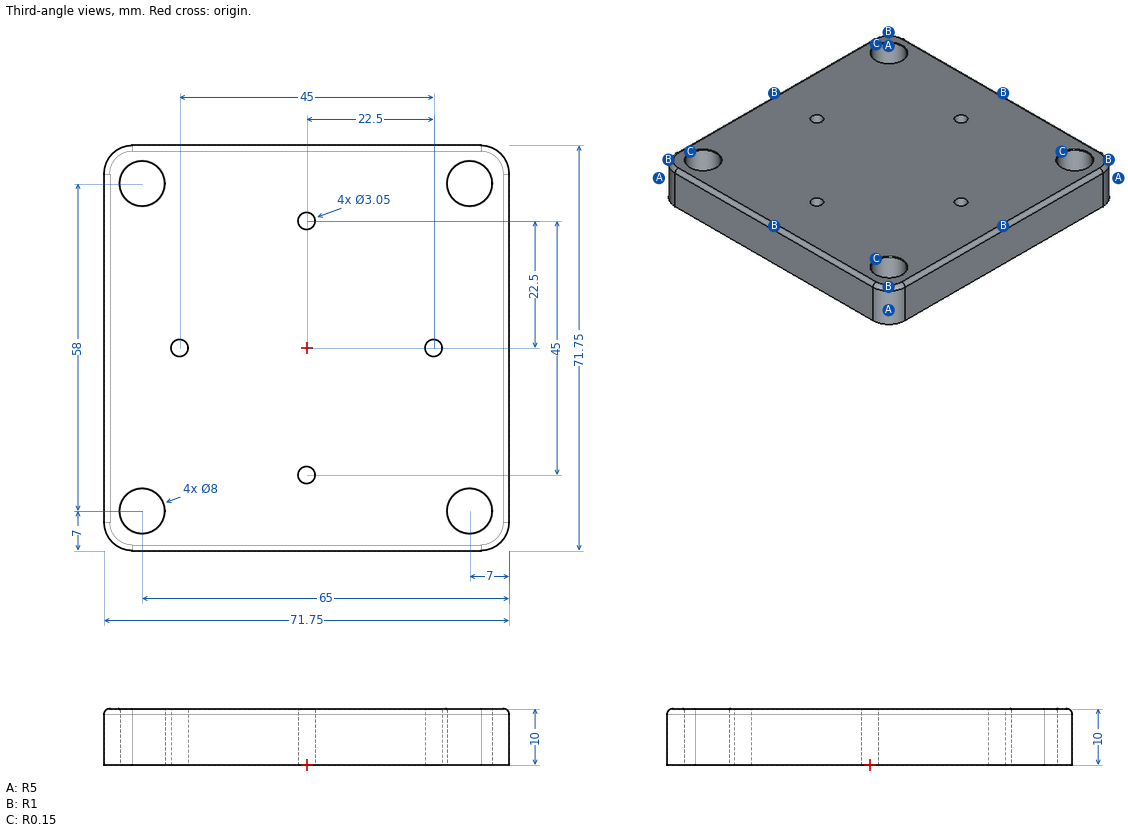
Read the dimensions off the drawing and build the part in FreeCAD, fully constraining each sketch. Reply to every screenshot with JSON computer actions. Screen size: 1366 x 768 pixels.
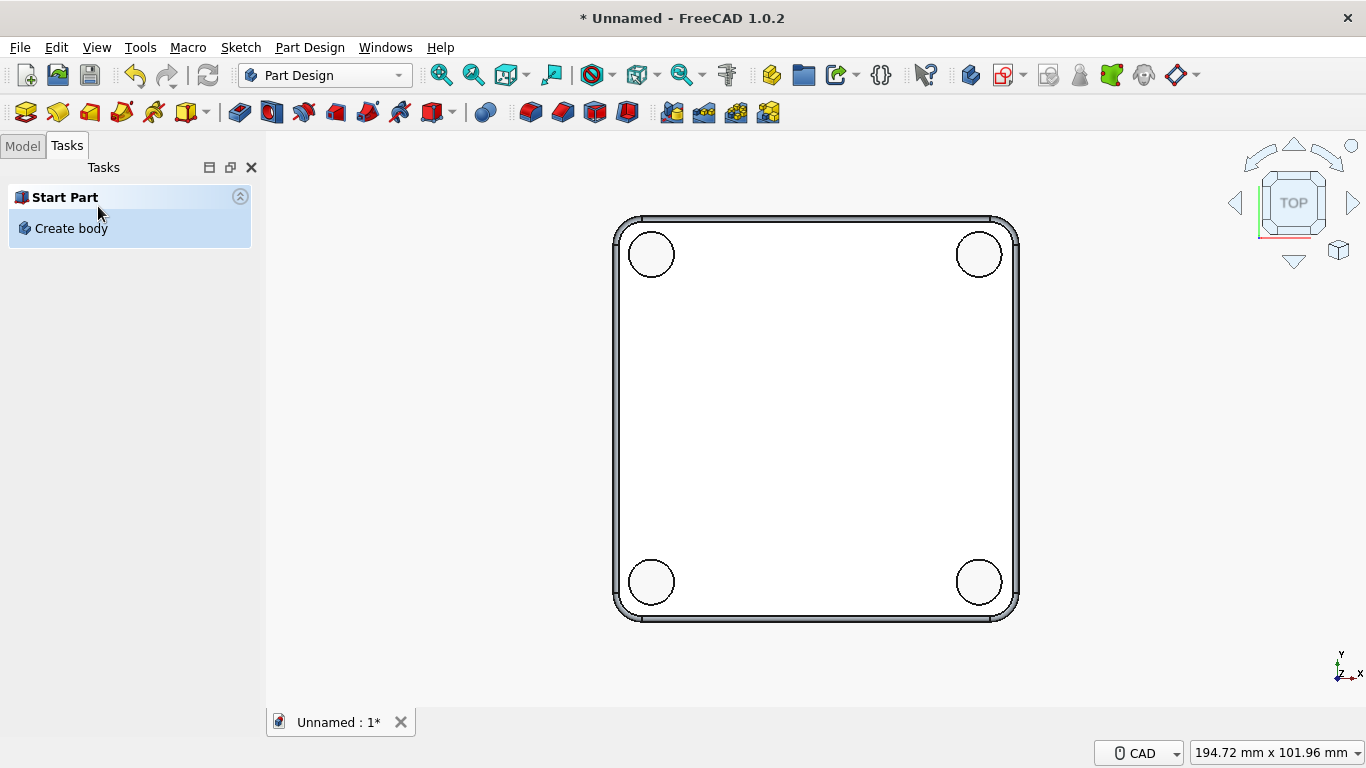
{"action": "left_click", "coordinate": [629, 253]}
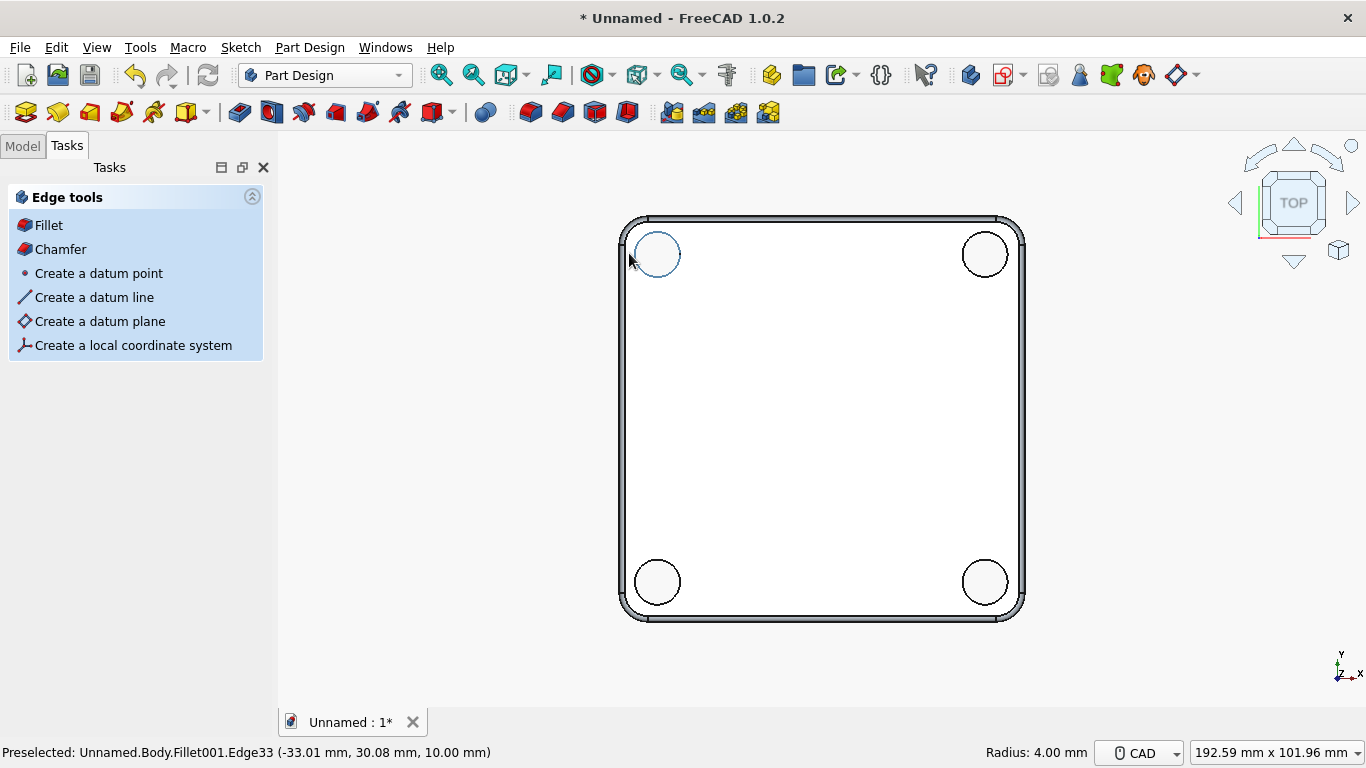
{"action": "left_click", "coordinate": [963, 253], "text": "ctrl"}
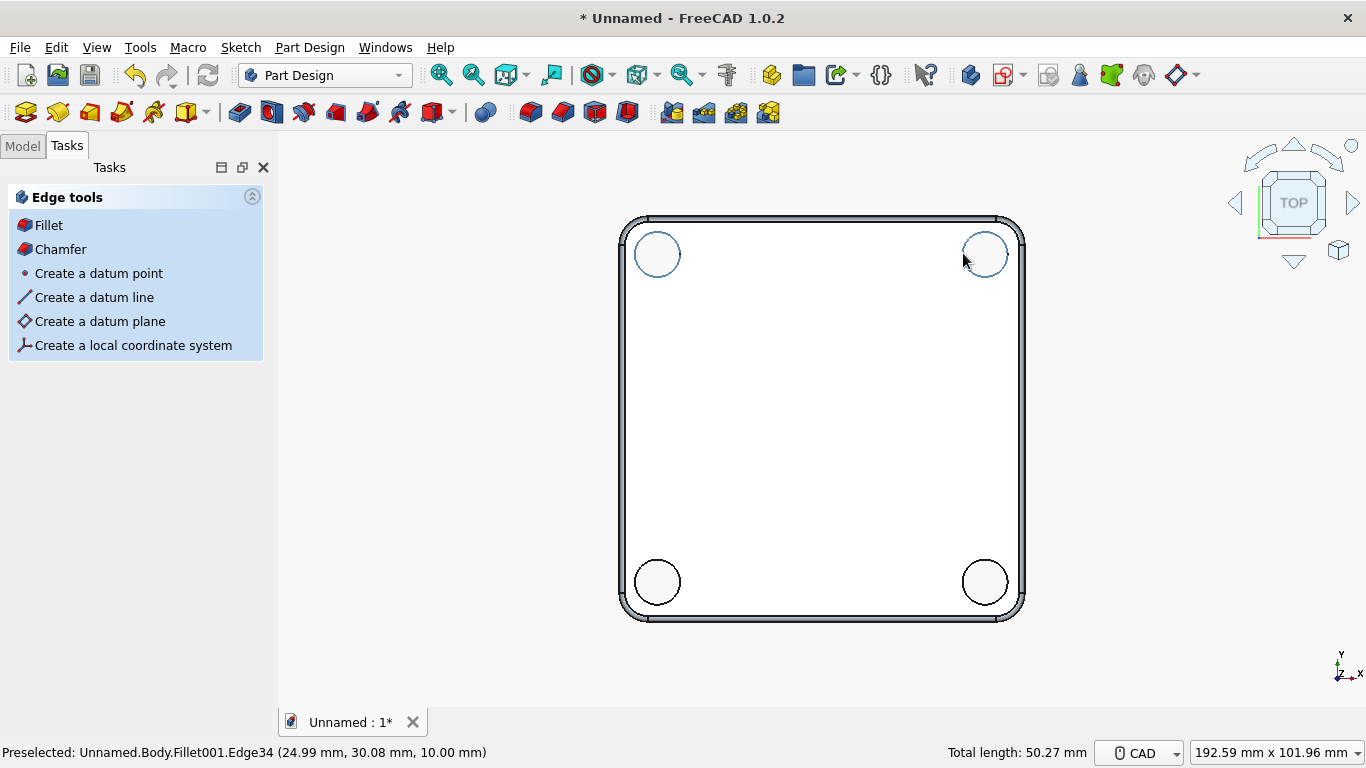
{"action": "left_click", "coordinate": [963, 581], "text": "ctrl"}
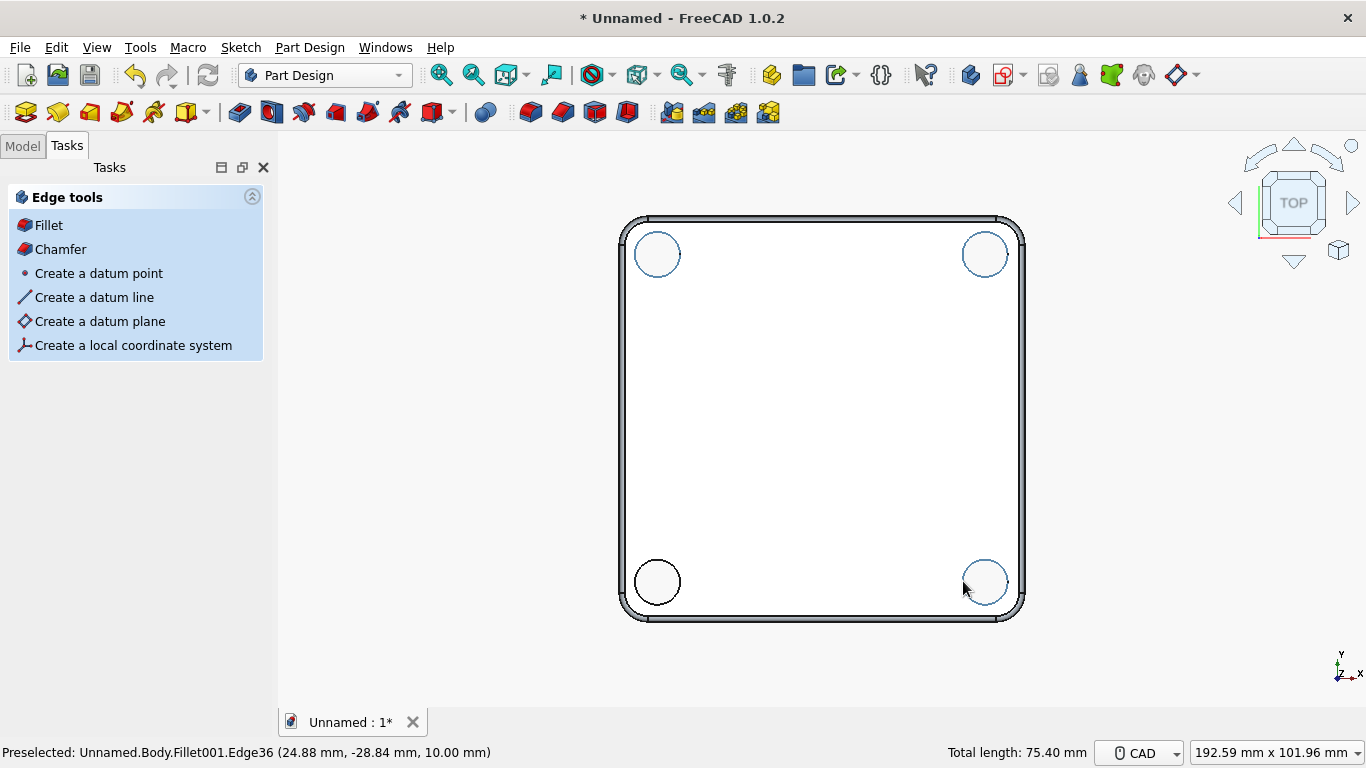
{"action": "left_click", "coordinate": [635, 581], "text": "ctrl"}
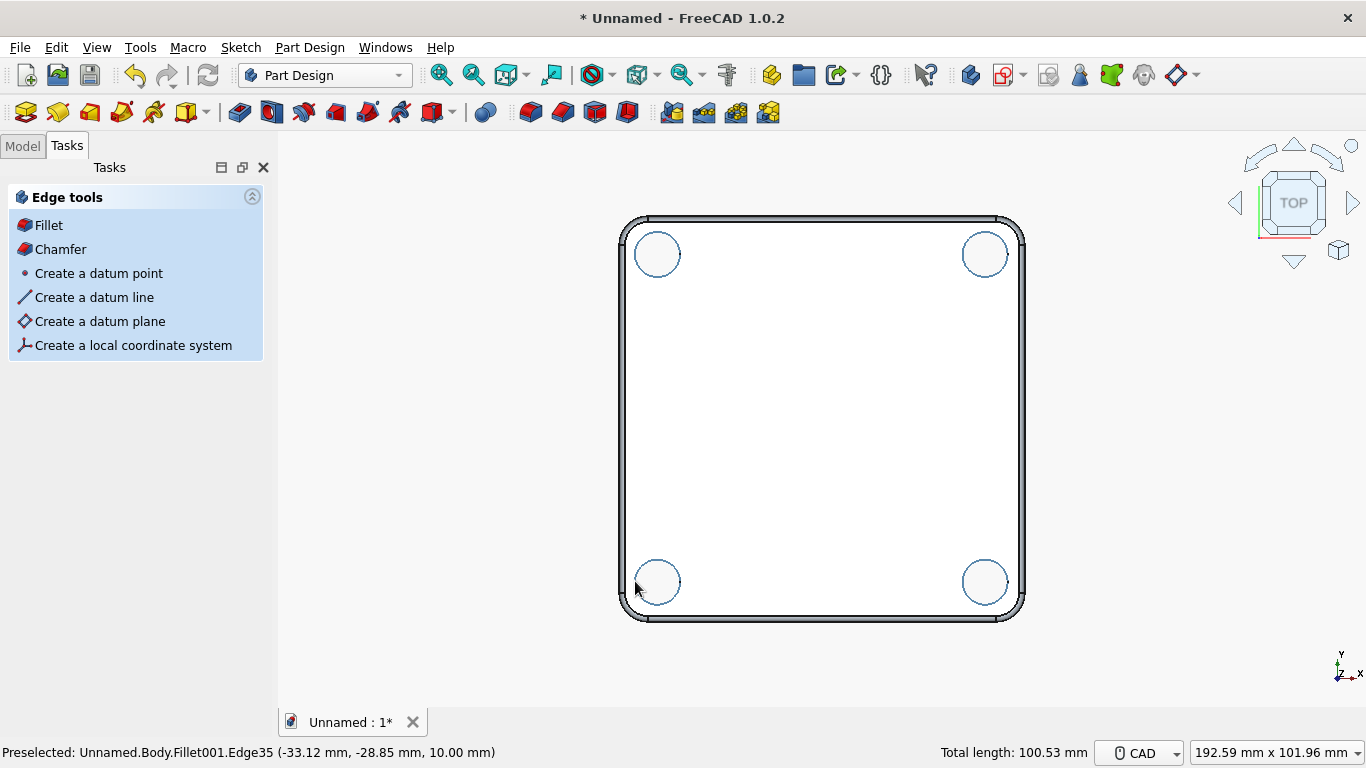
{"action": "left_click", "coordinate": [532, 112]}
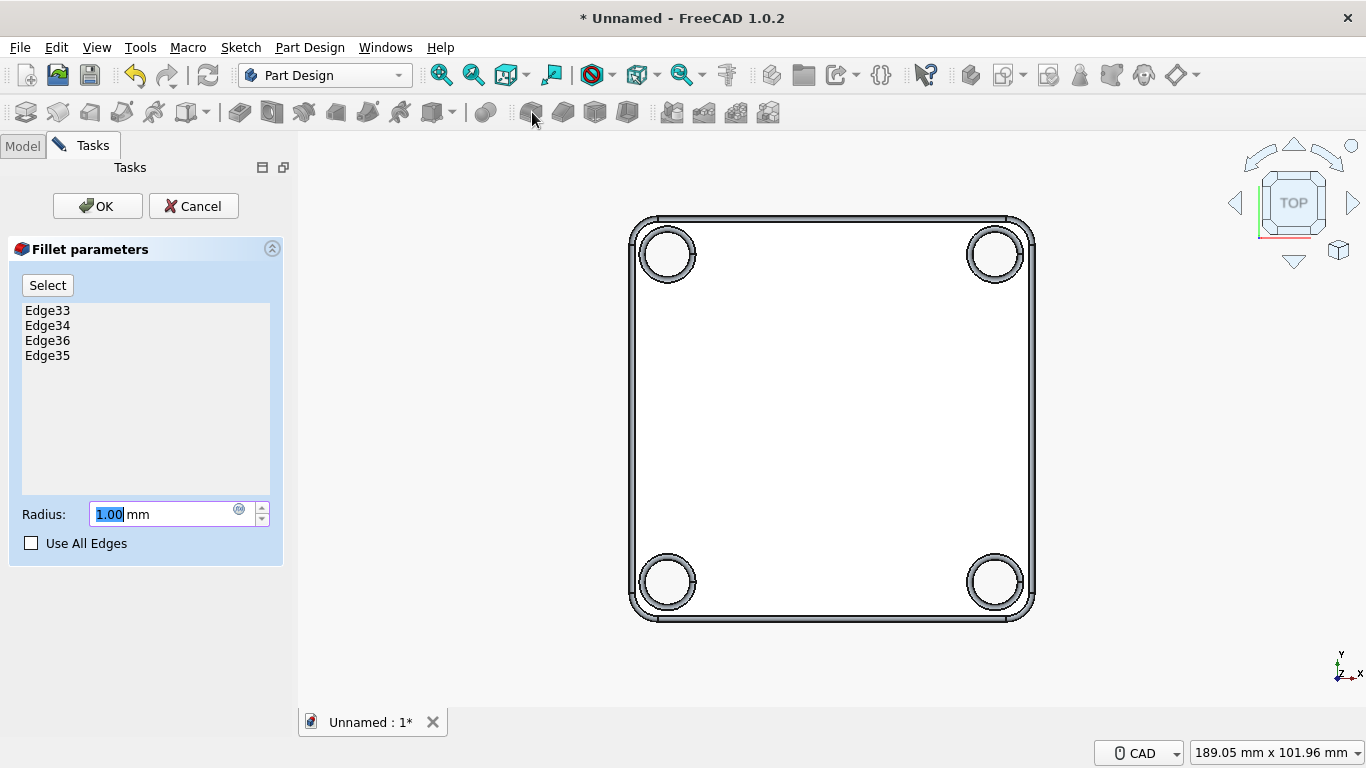
{"action": "type", "text": "0.15"}
{"action": "key", "text": "Tab"}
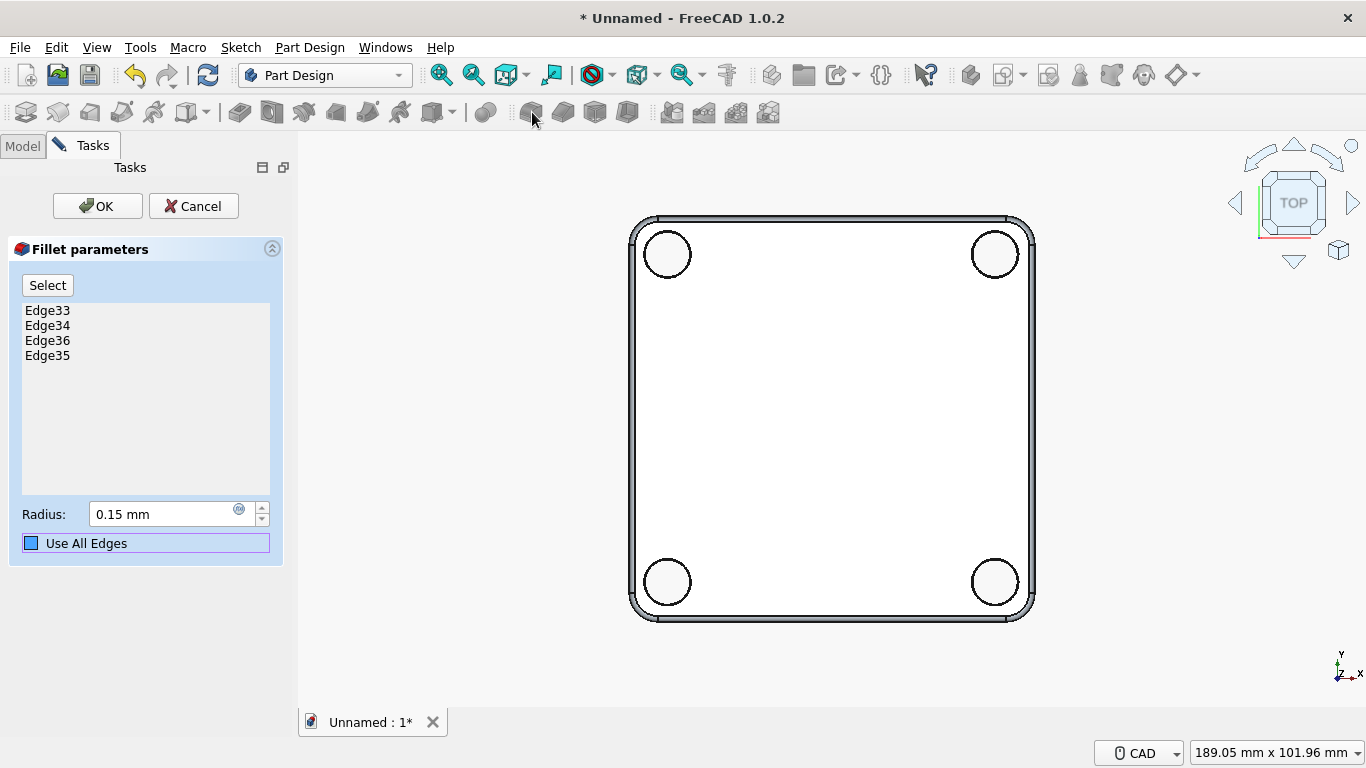
{"action": "left_click", "coordinate": [98, 206]}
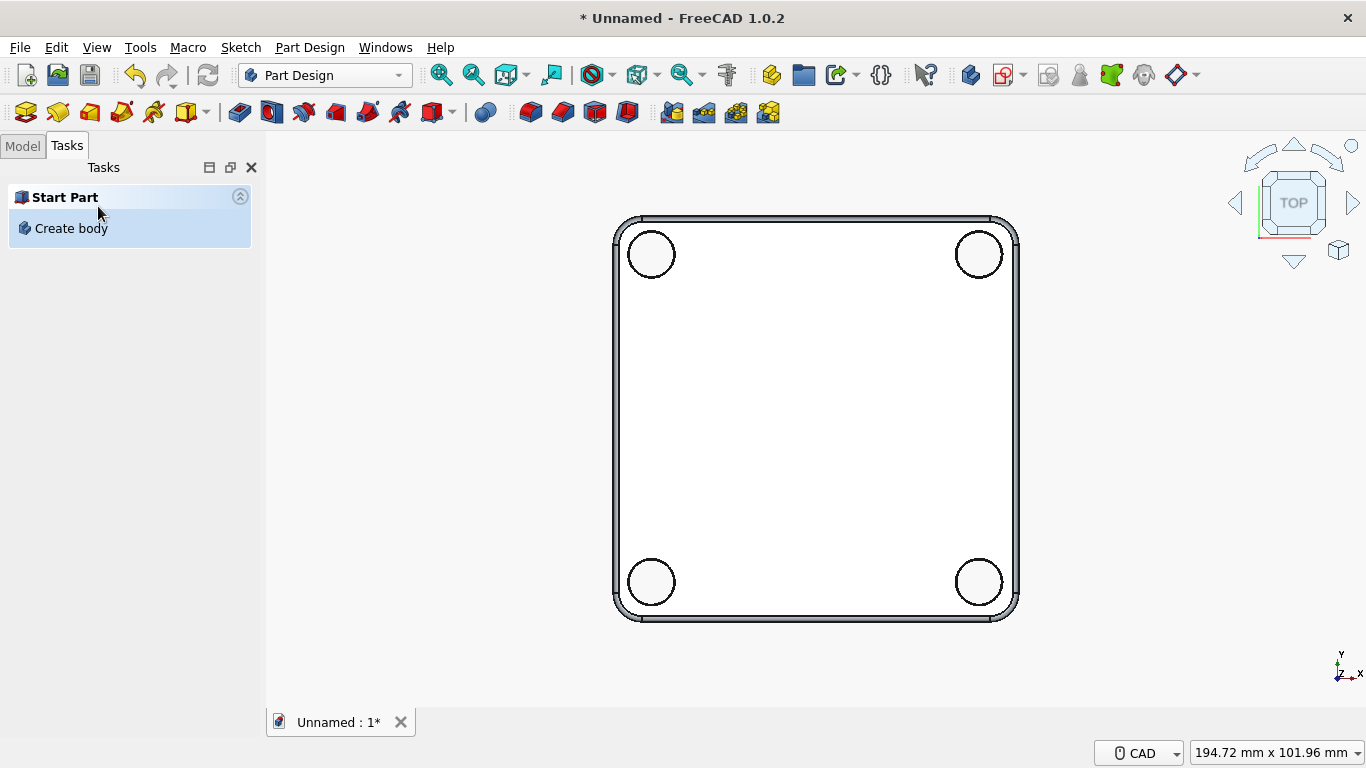
{"action": "left_click", "coordinate": [816, 418]}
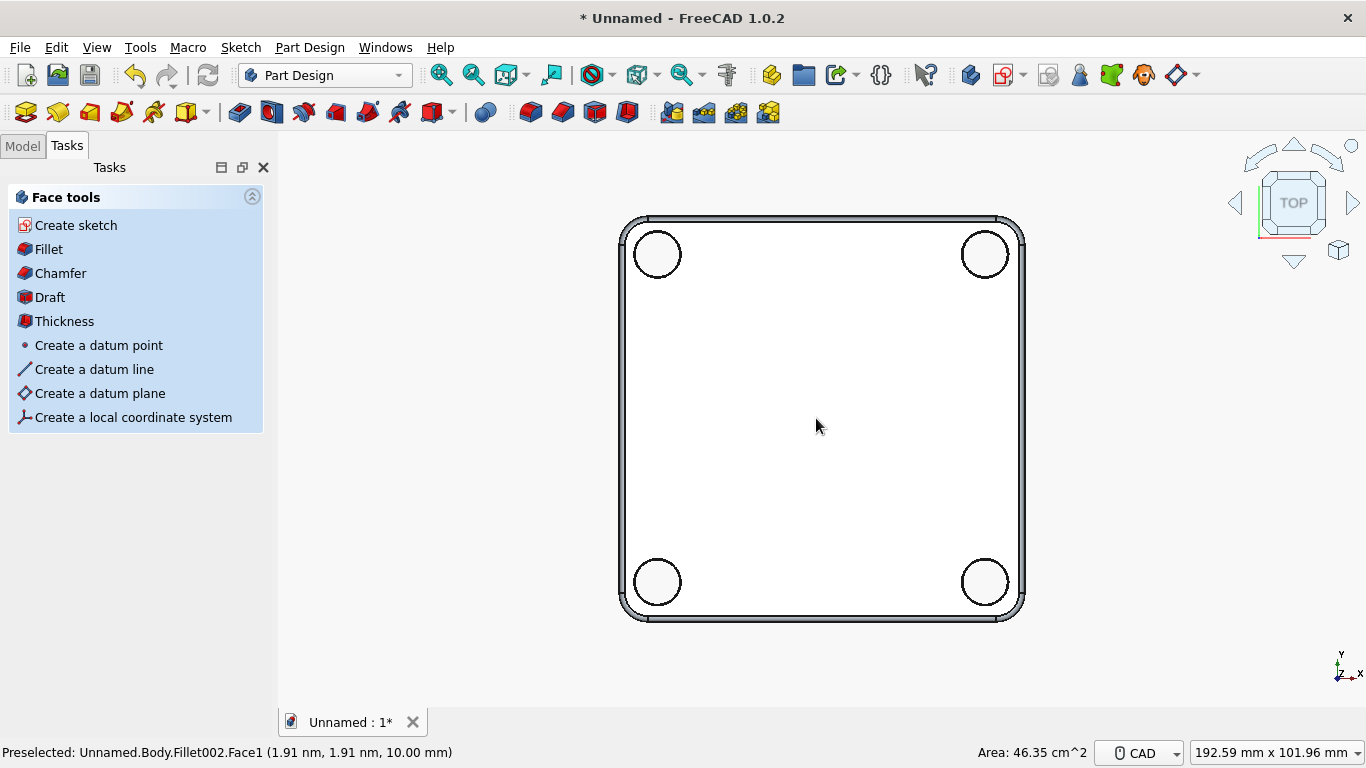
{"action": "left_click", "coordinate": [1004, 76]}